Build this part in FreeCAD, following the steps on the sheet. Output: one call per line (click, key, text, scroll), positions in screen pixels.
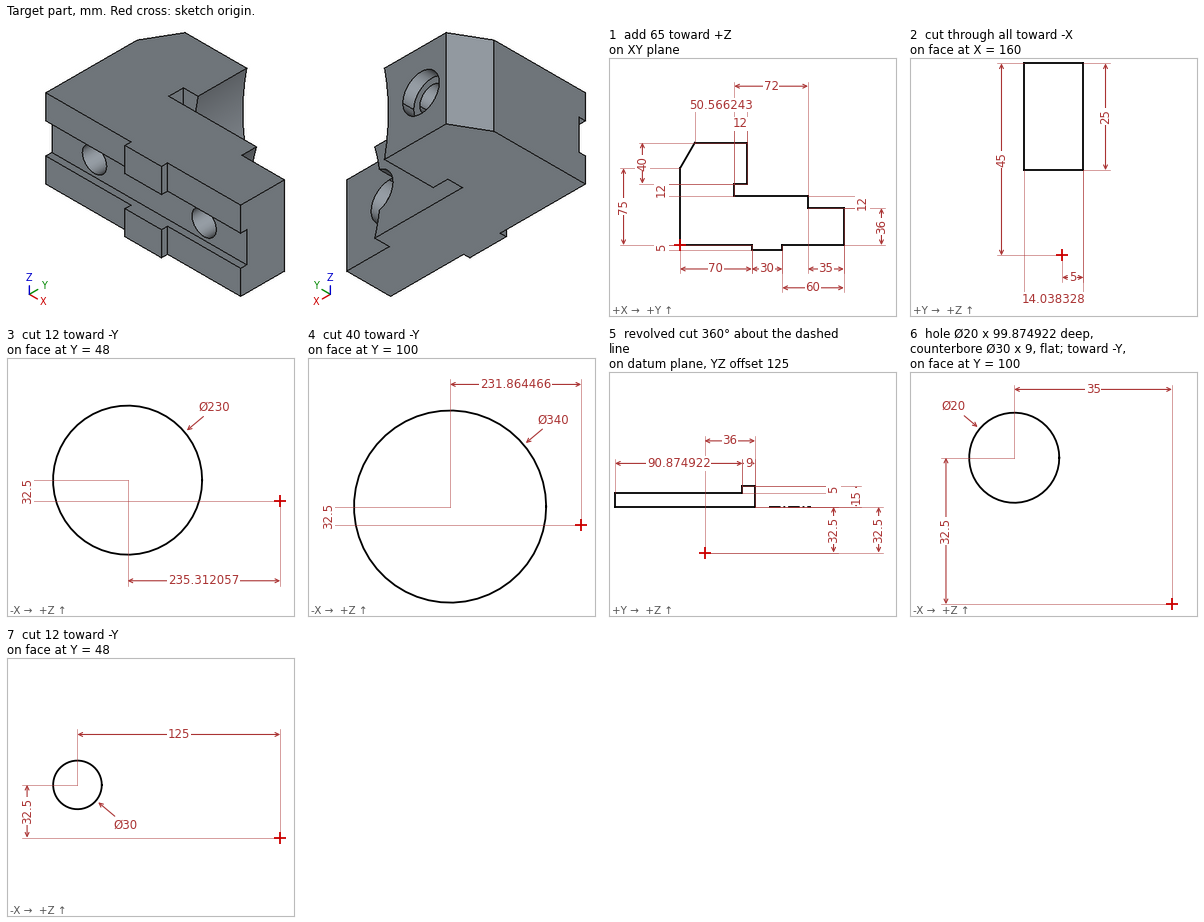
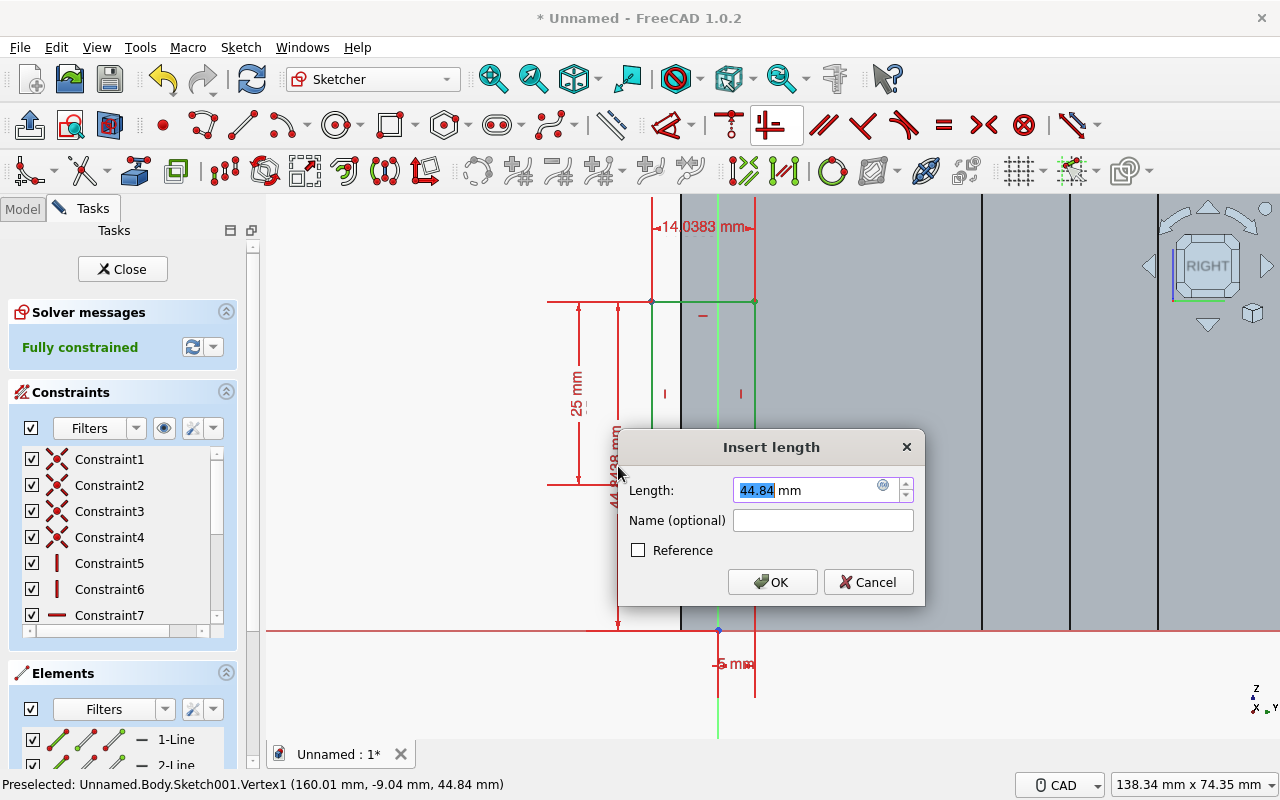
text(45)
key(Return)
key(Escape)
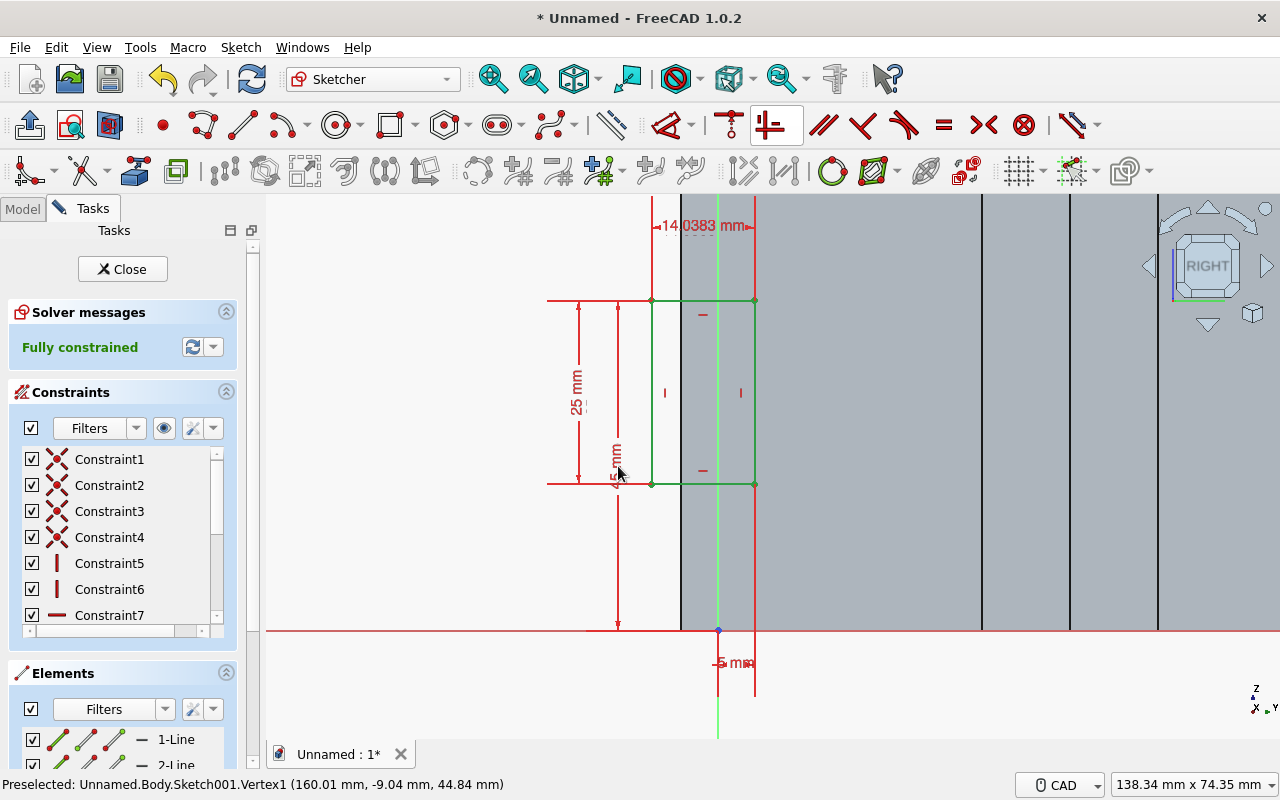
click(123, 269)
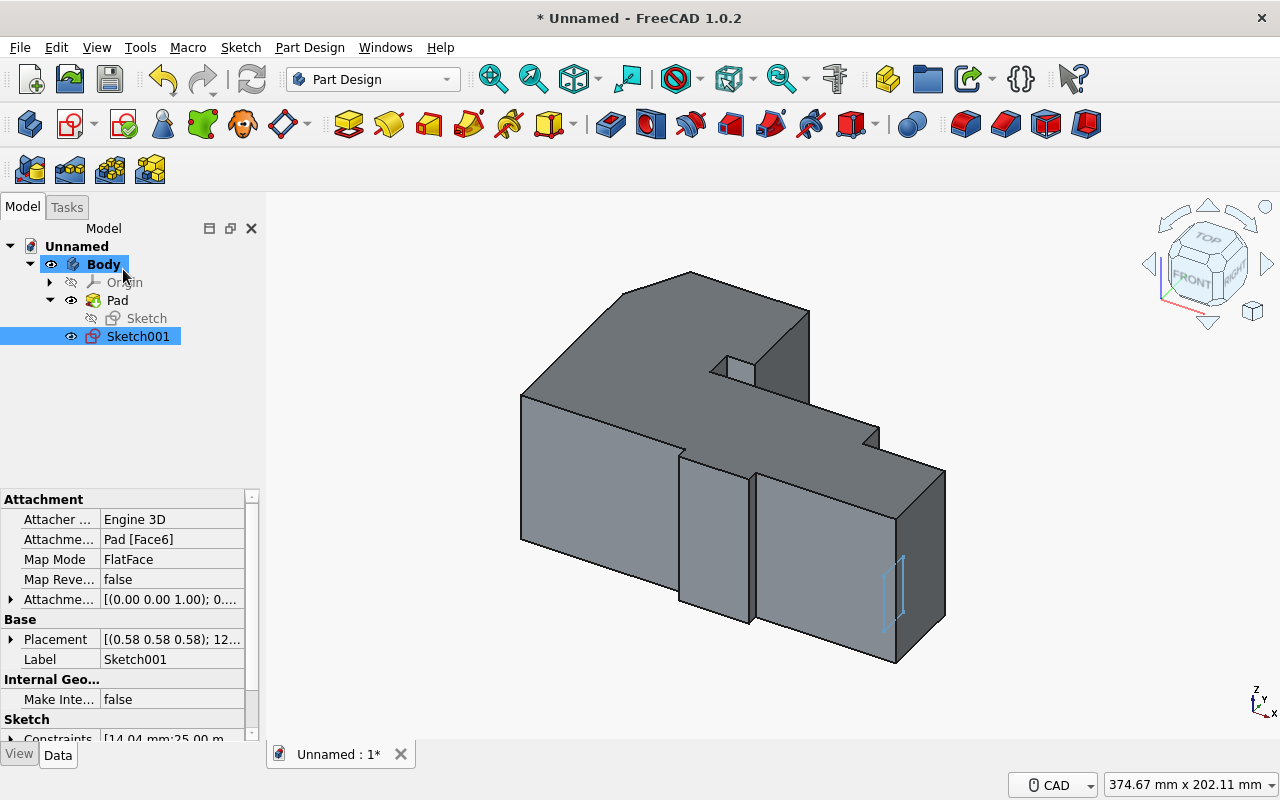
click(612, 124)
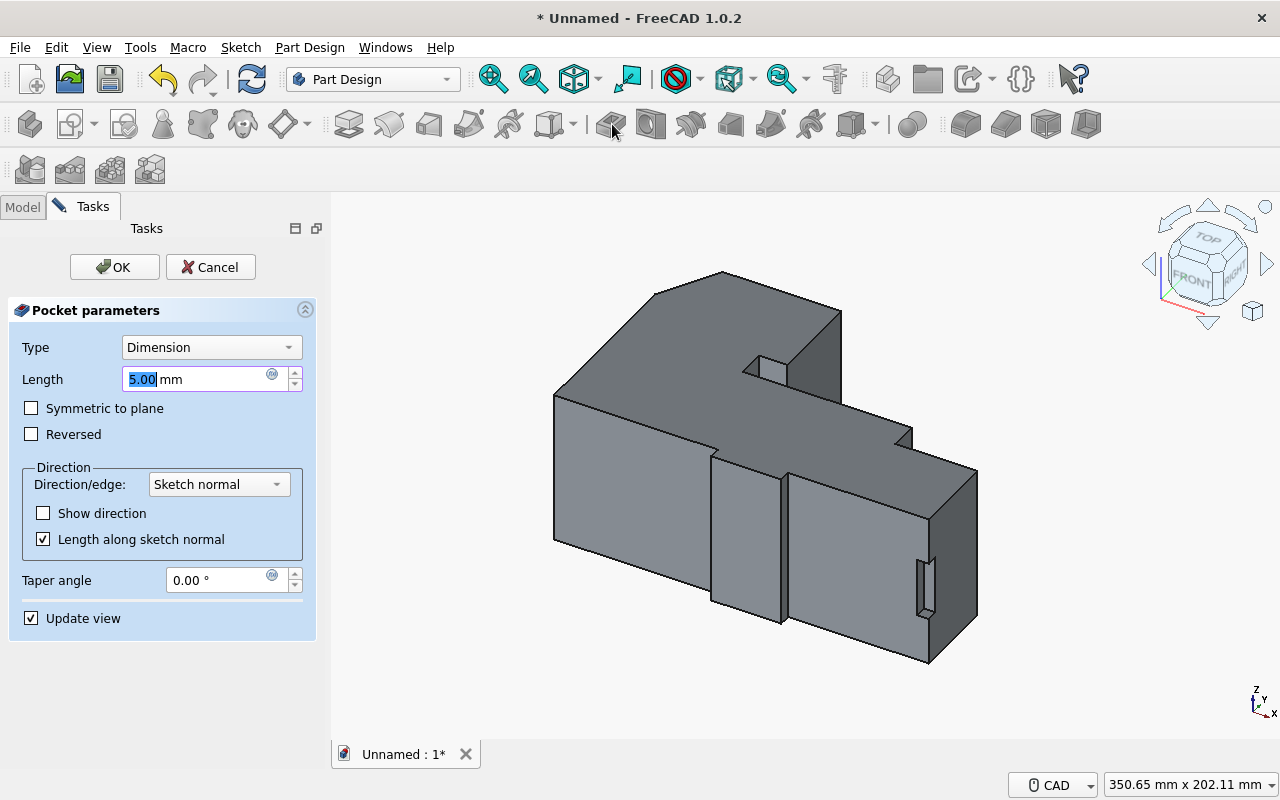
click(212, 348)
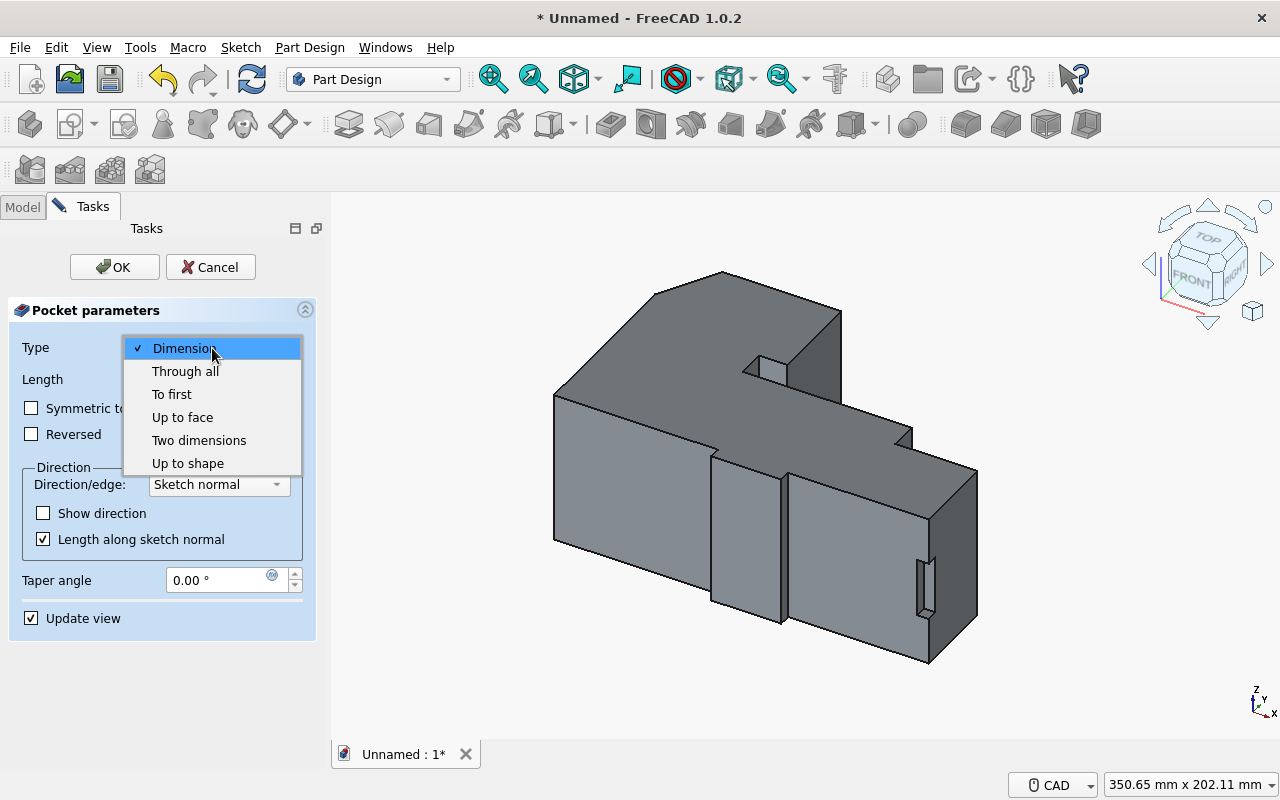
click(212, 372)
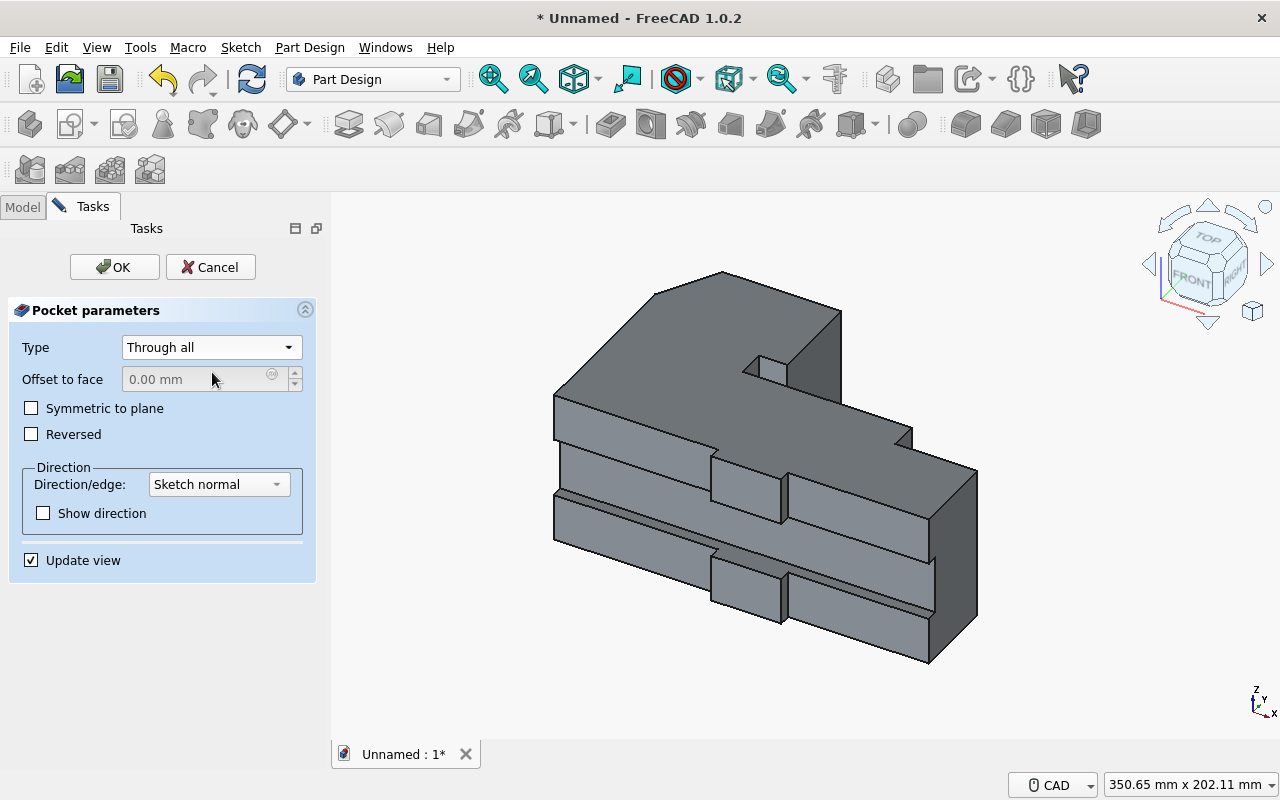
click(115, 267)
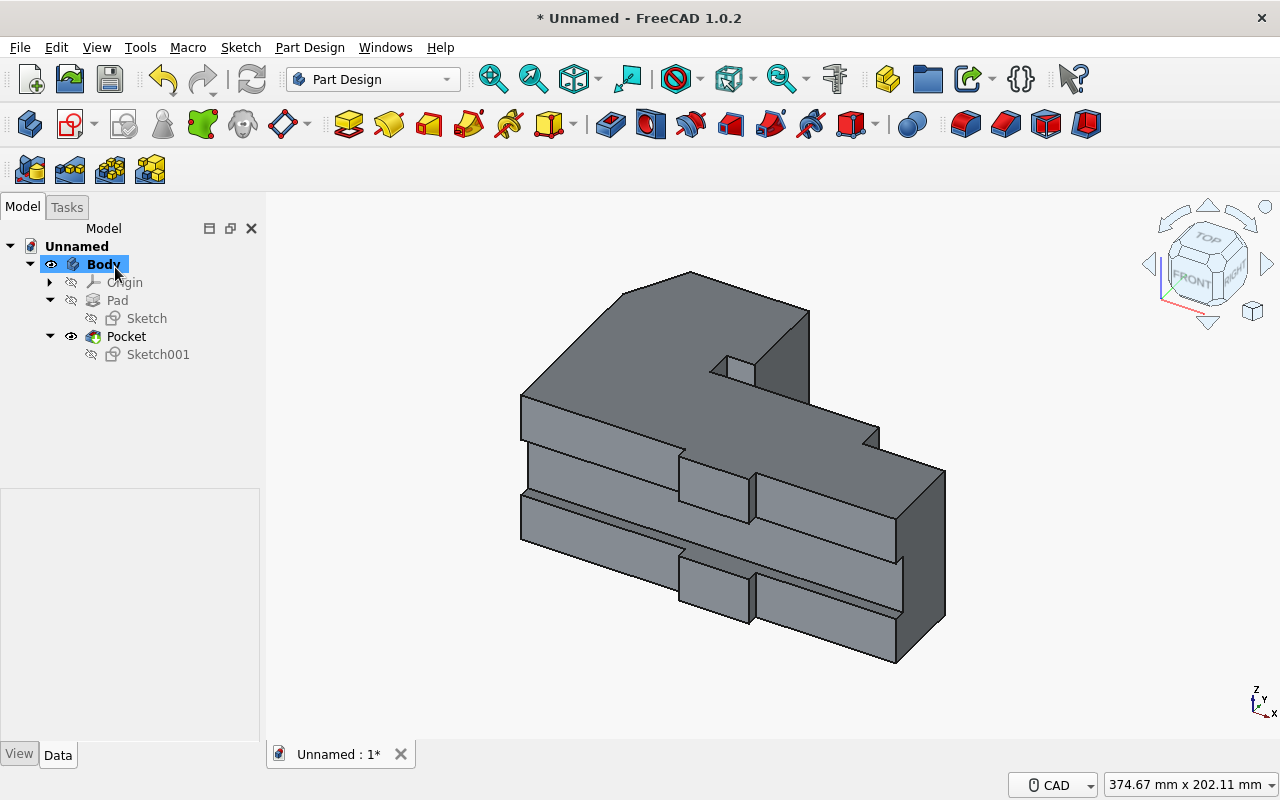
key(4)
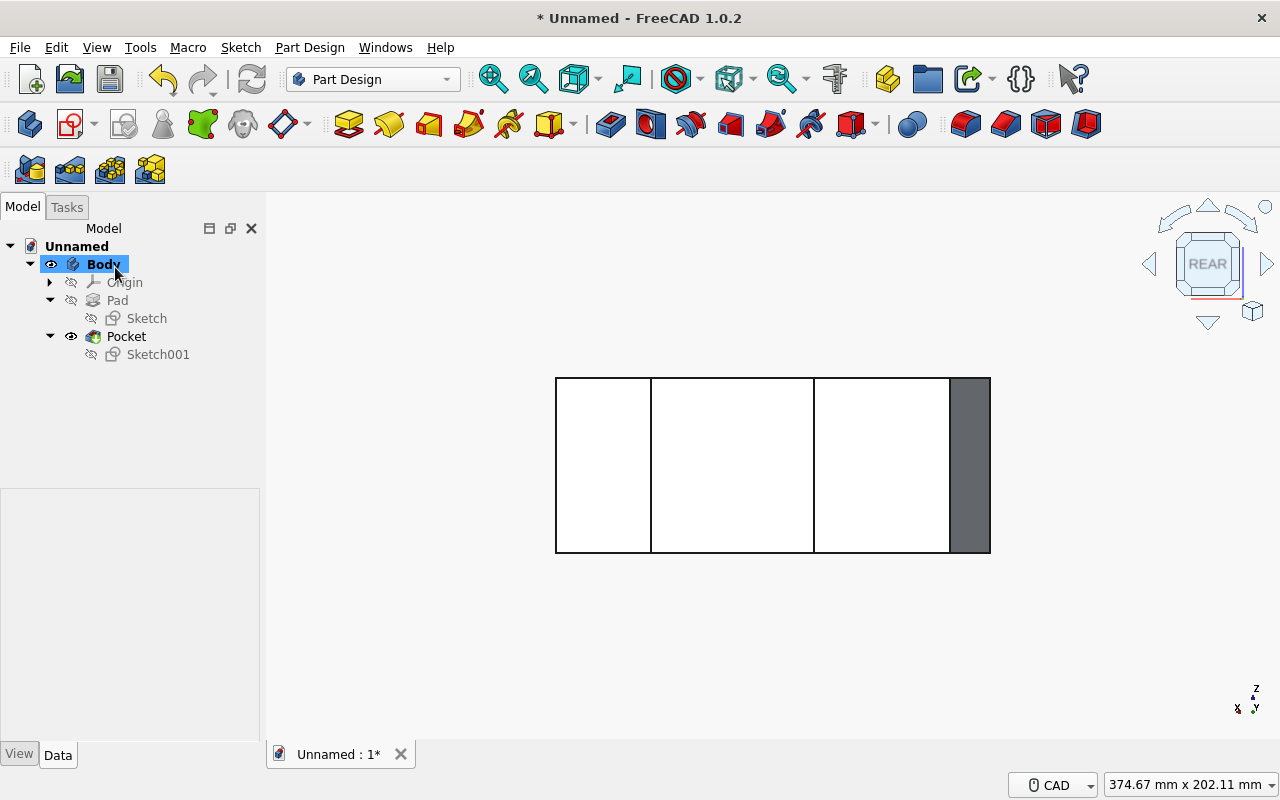
click(494, 80)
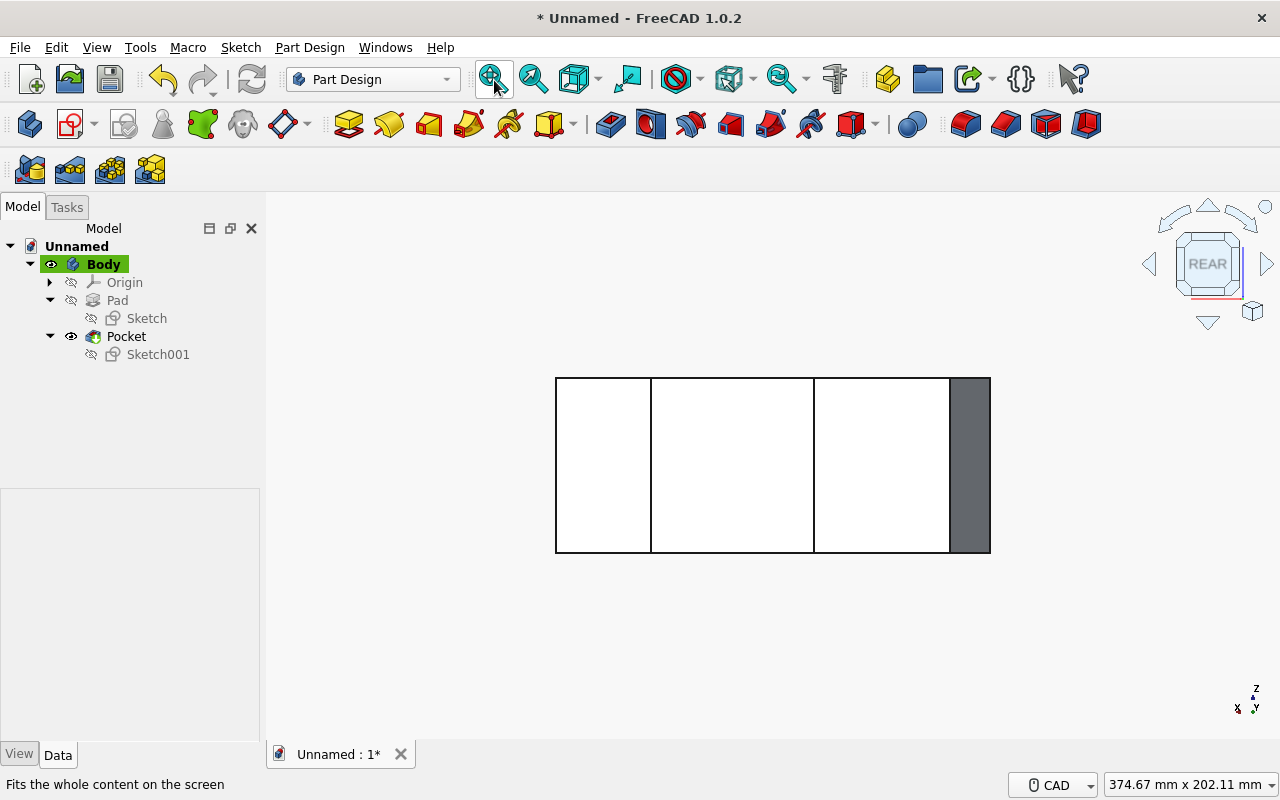
click(749, 465)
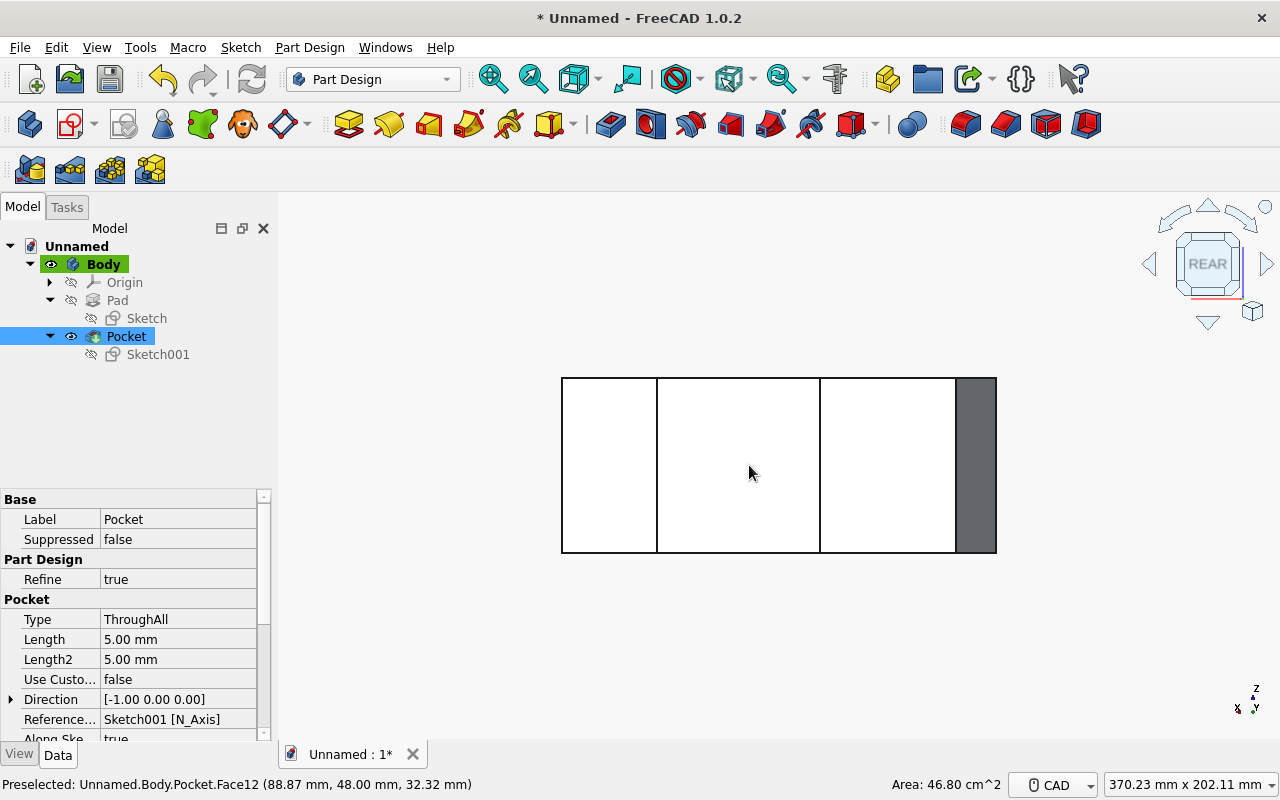
click(70, 124)